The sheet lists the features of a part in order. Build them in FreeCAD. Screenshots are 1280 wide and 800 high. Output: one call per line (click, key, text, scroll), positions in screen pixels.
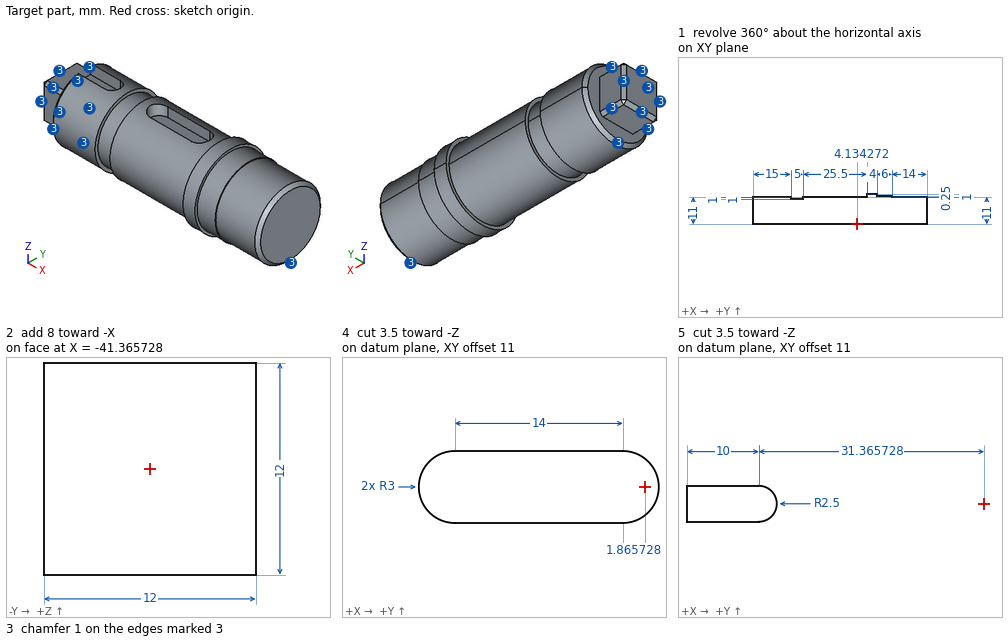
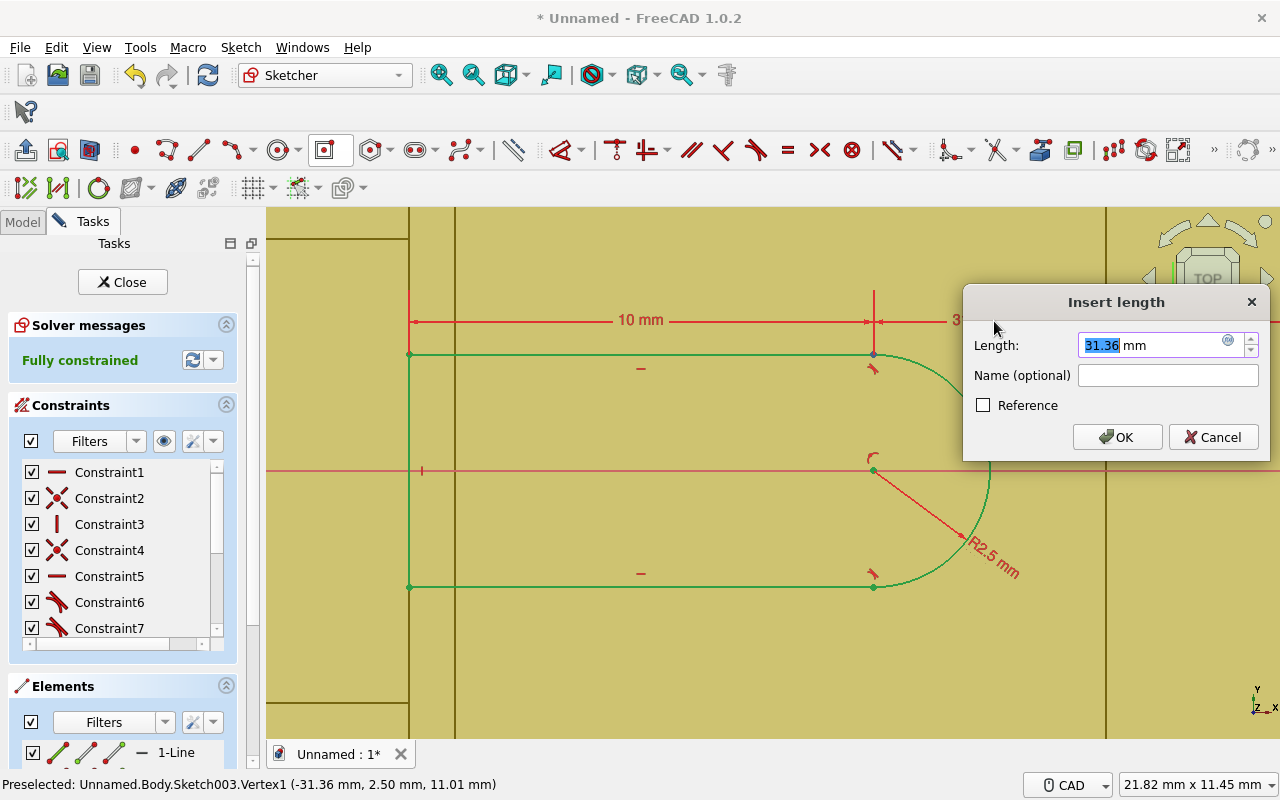
text(31.365728)
key(Return)
key(Escape)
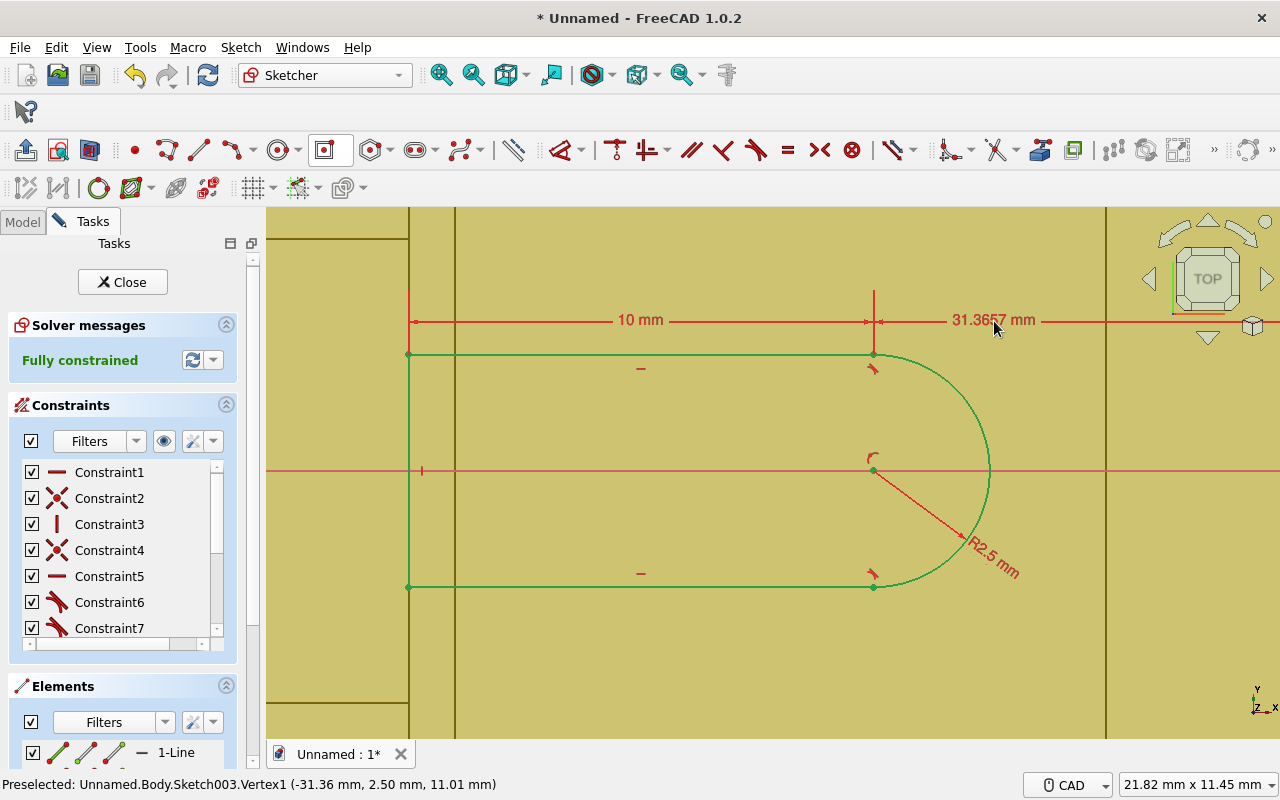
click(123, 282)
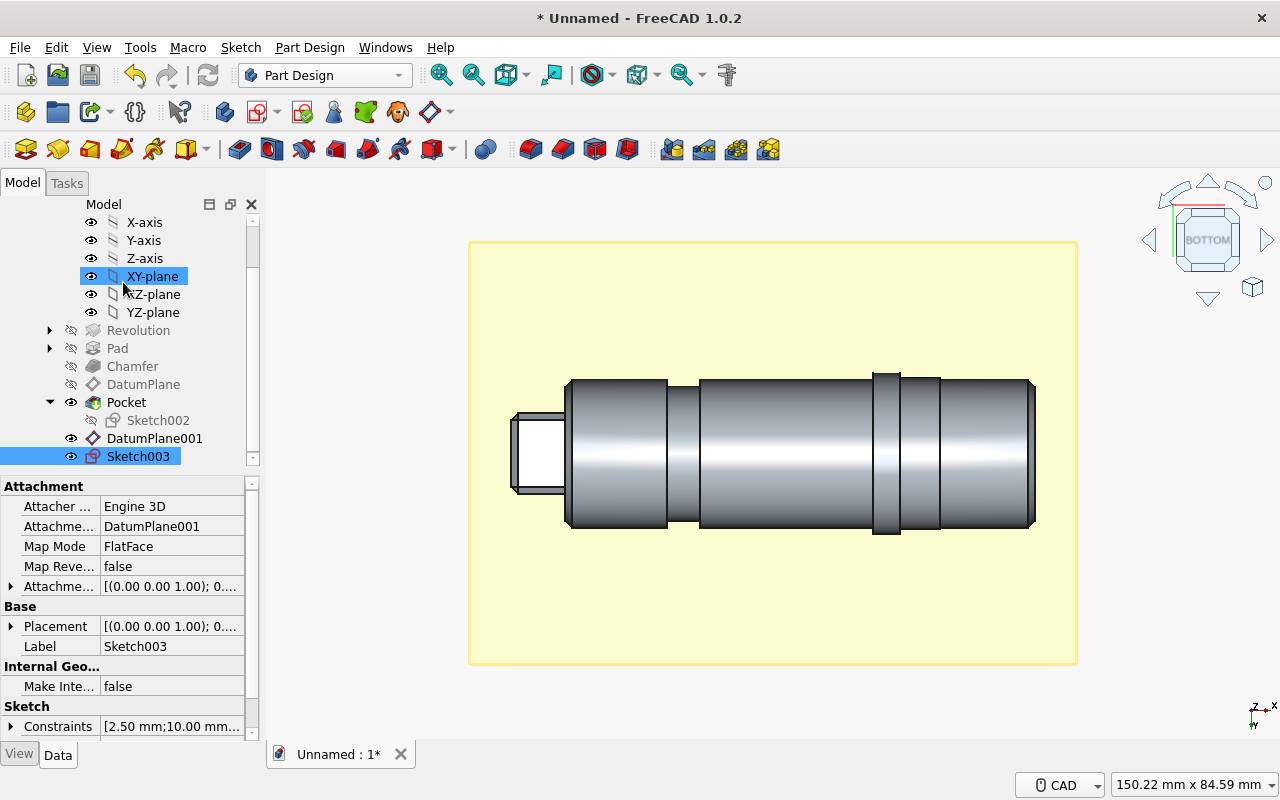
click(240, 150)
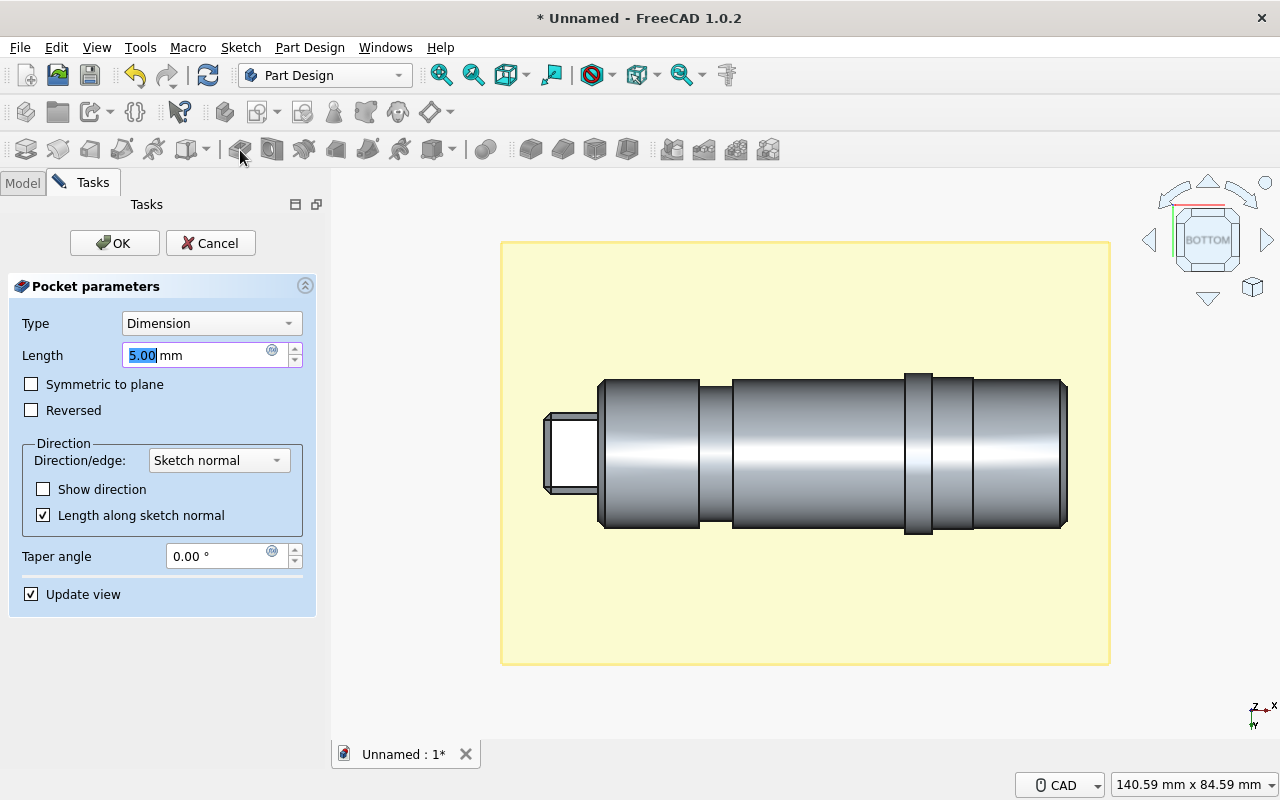
text(3.5)
key(Tab)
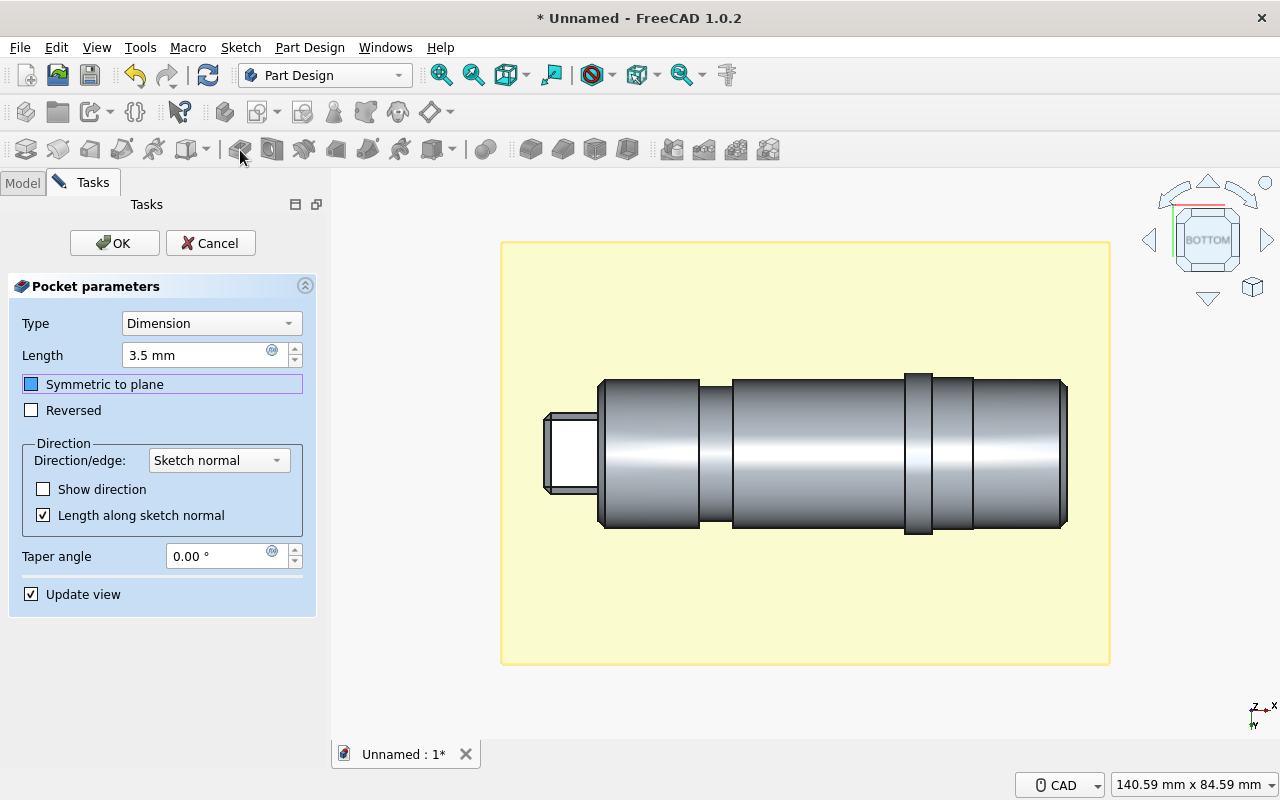
click(115, 243)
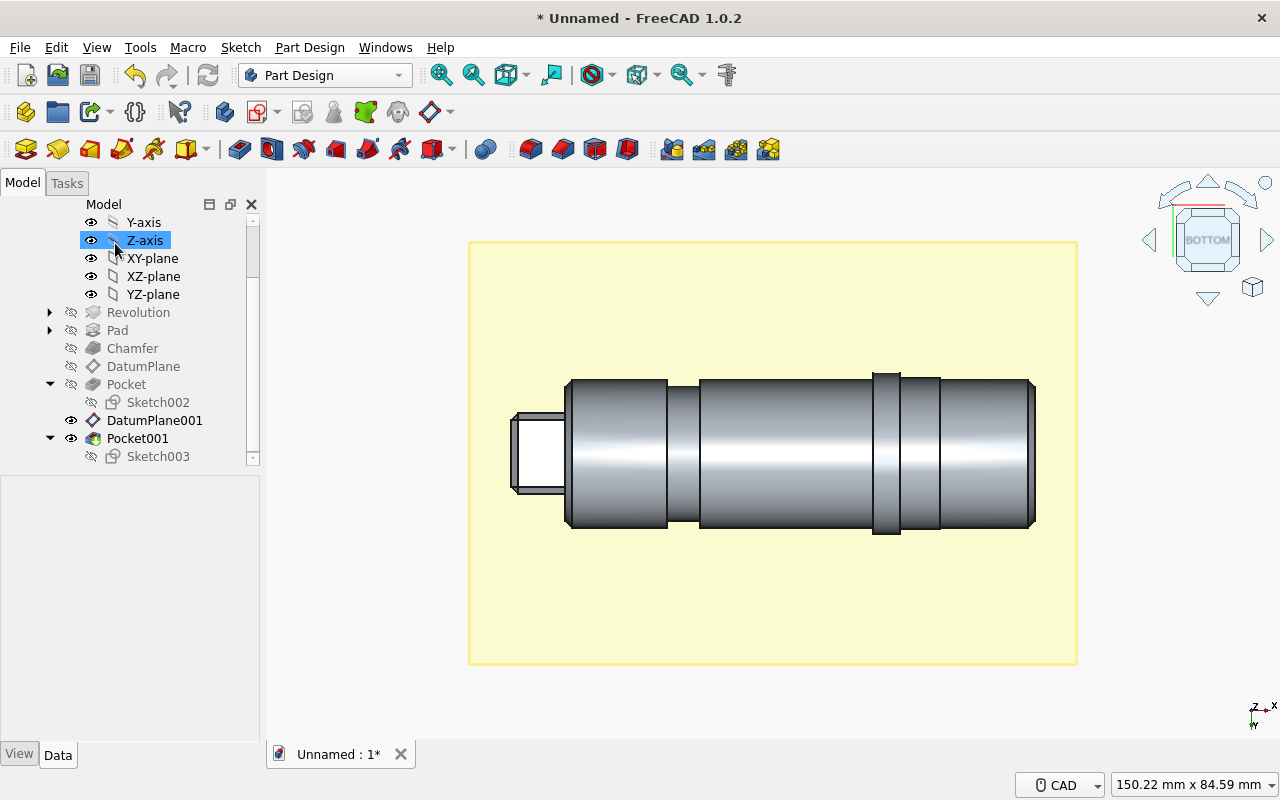
click(116, 420)
key(space)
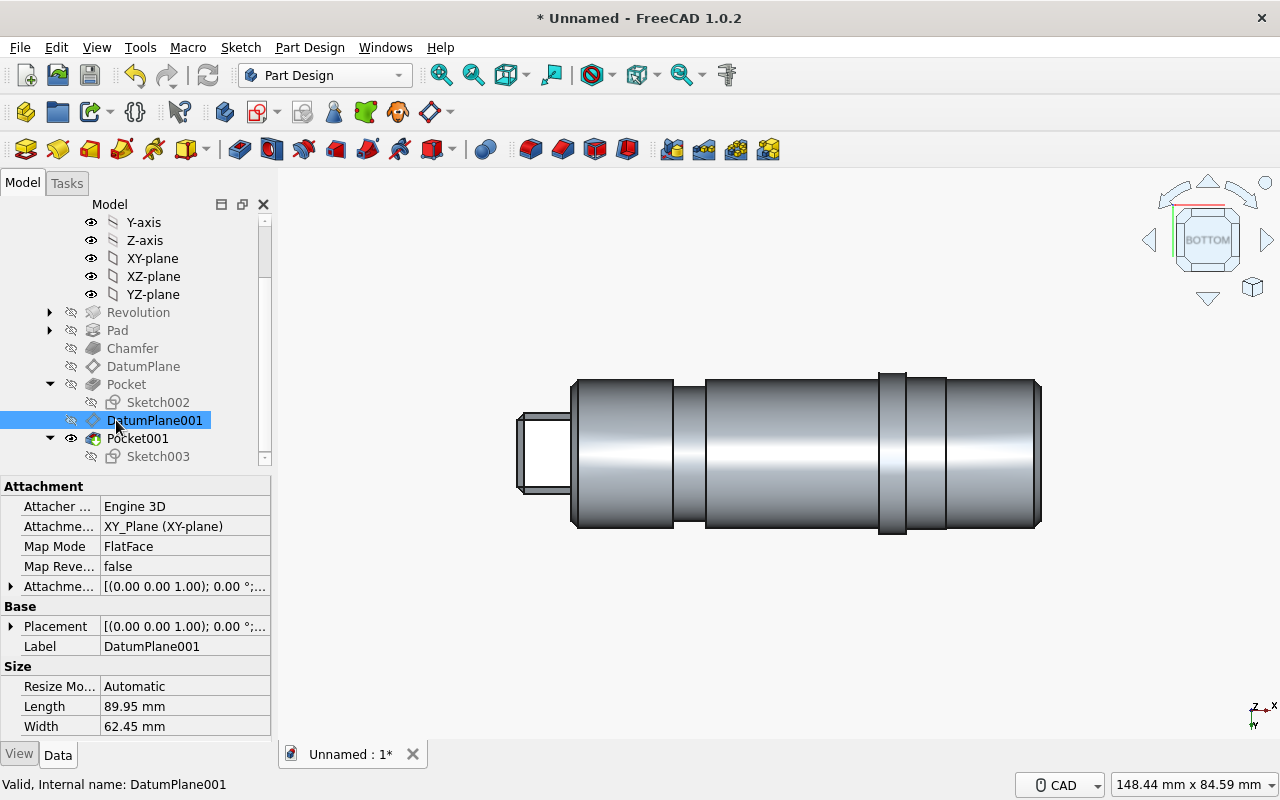
key(0)